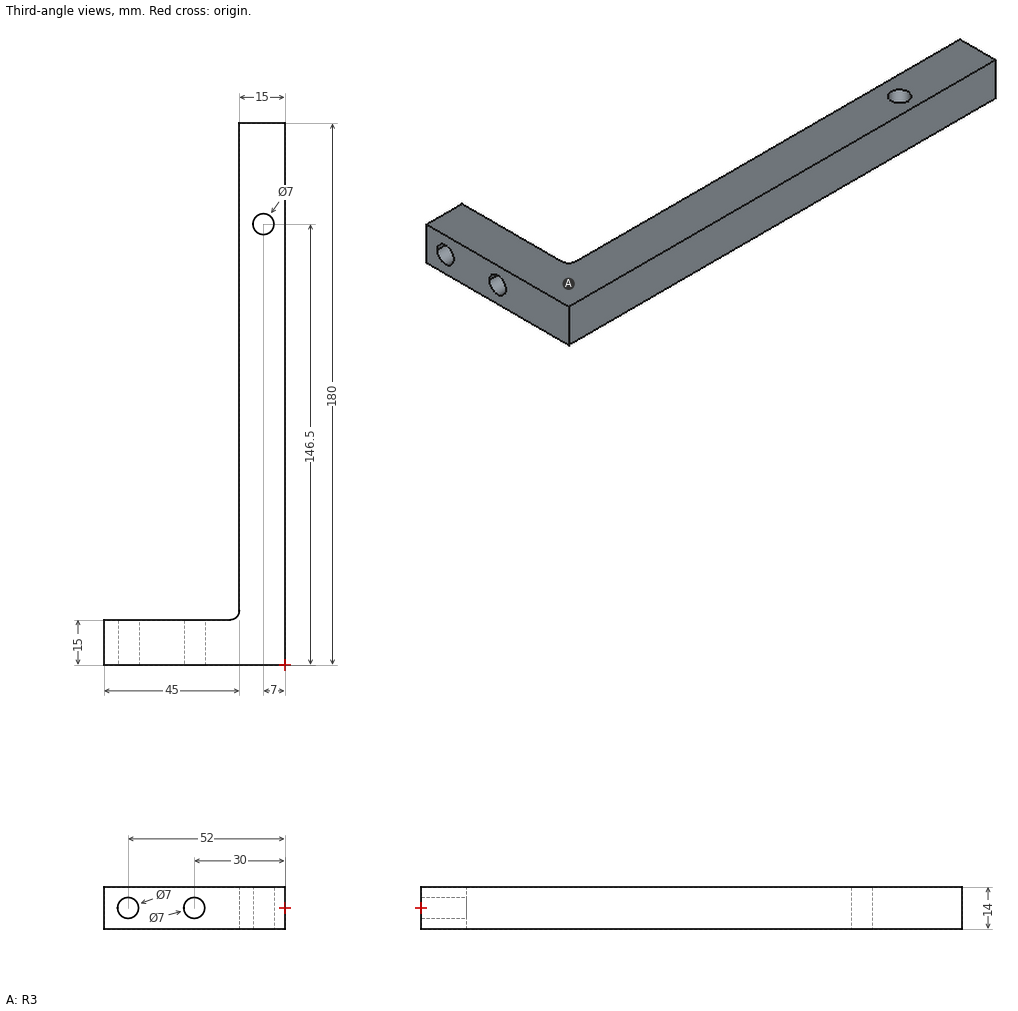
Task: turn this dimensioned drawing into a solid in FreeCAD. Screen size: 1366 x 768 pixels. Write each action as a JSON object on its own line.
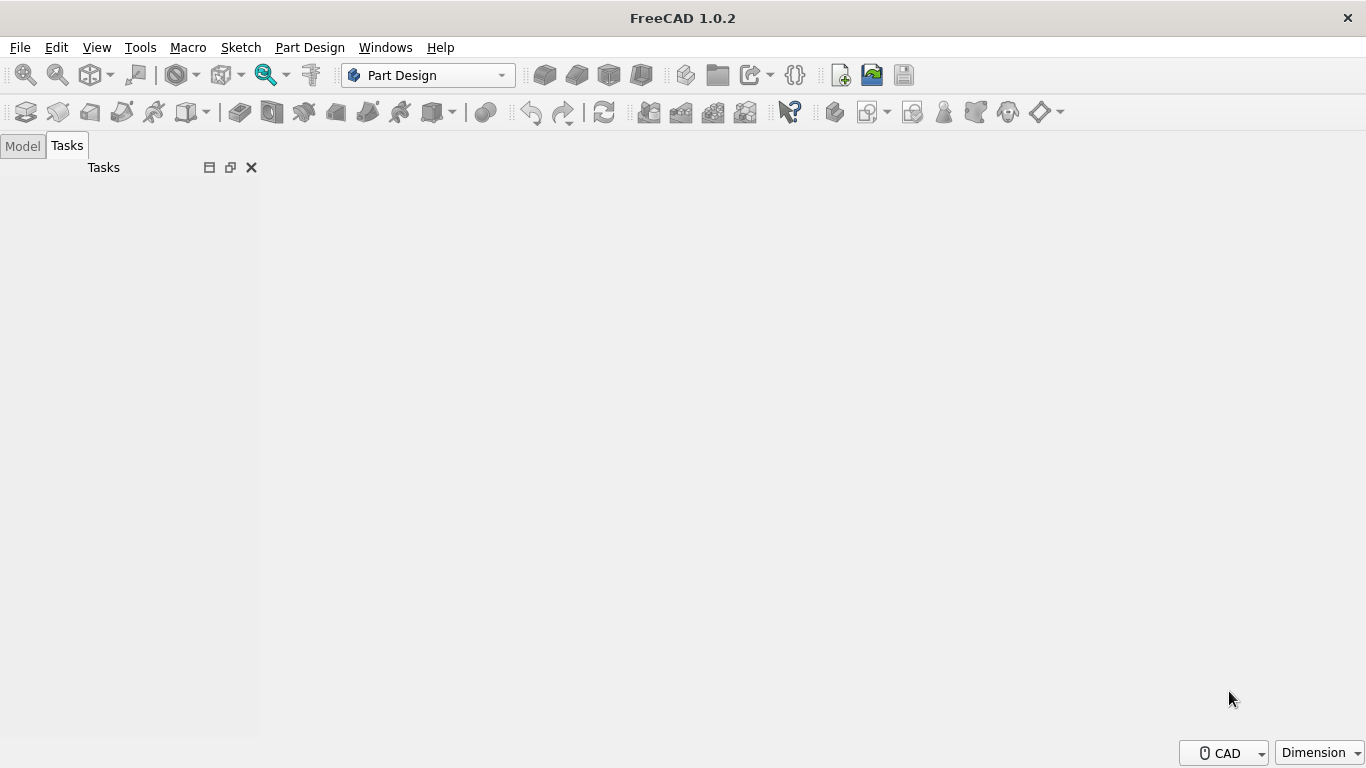
{"action": "left_click", "coordinate": [840, 76]}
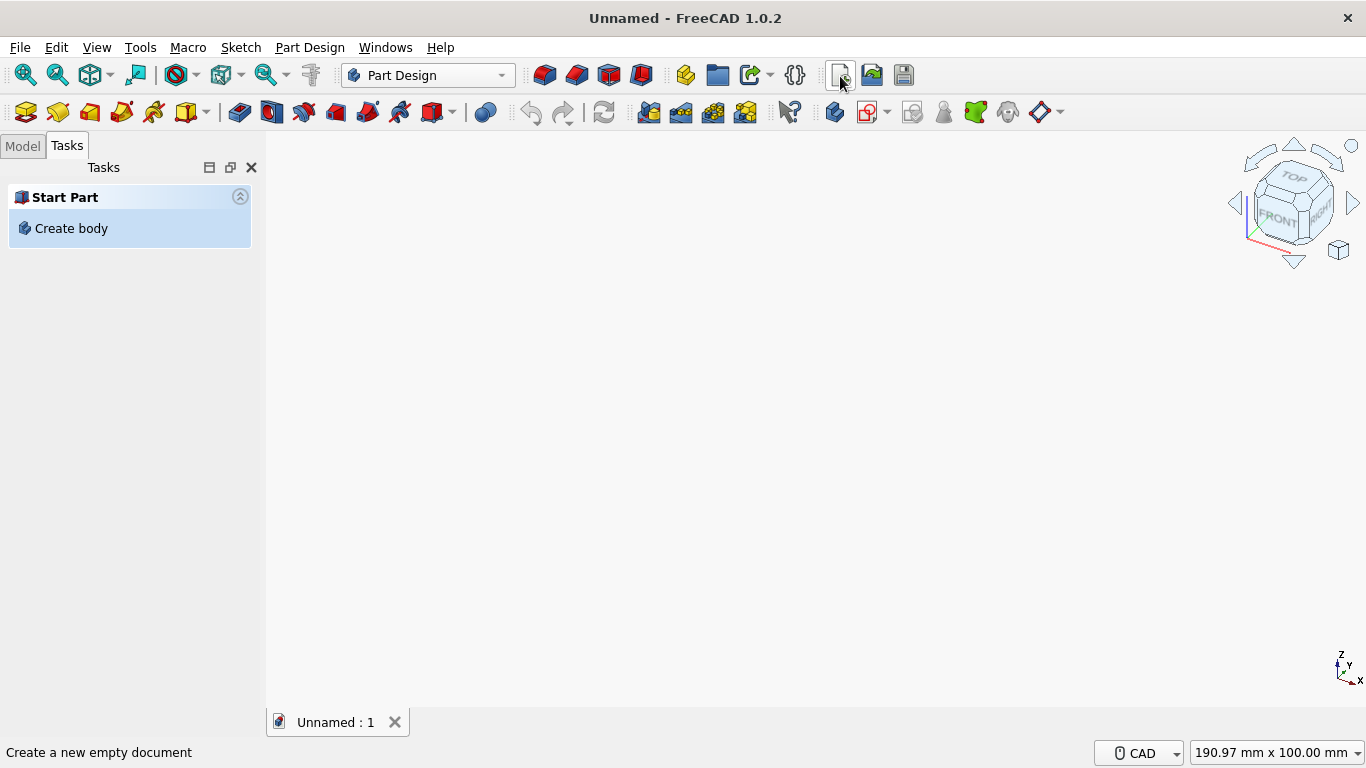
{"action": "left_click", "coordinate": [868, 112]}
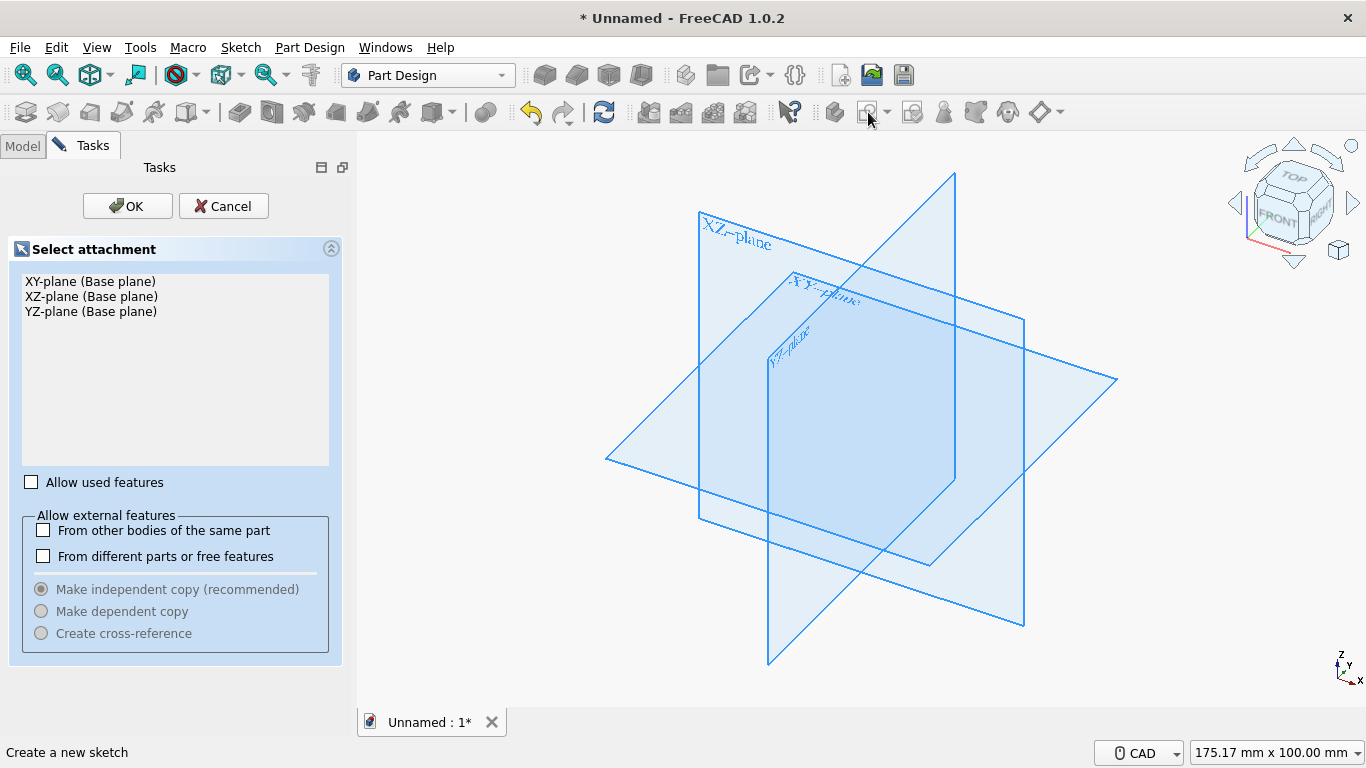
{"action": "left_click", "coordinate": [82, 282]}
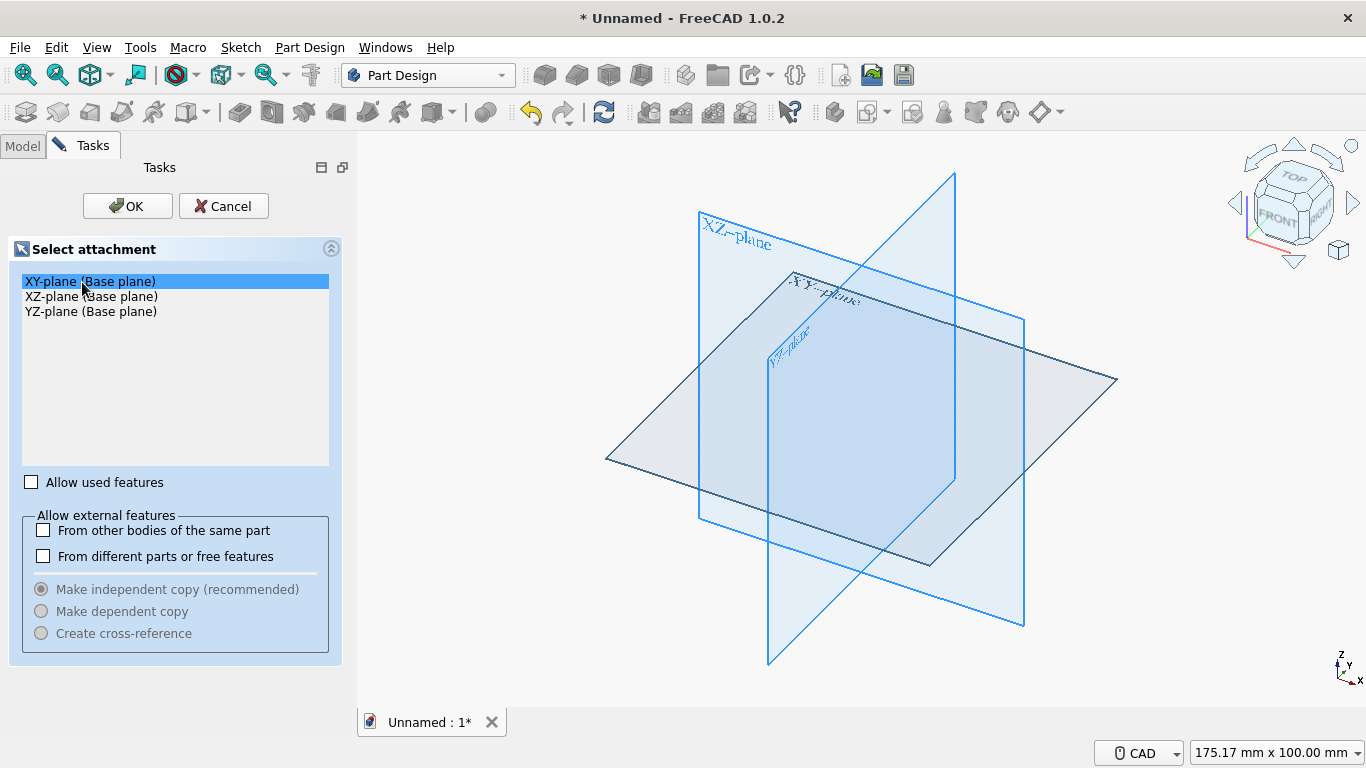
{"action": "left_click", "coordinate": [128, 206]}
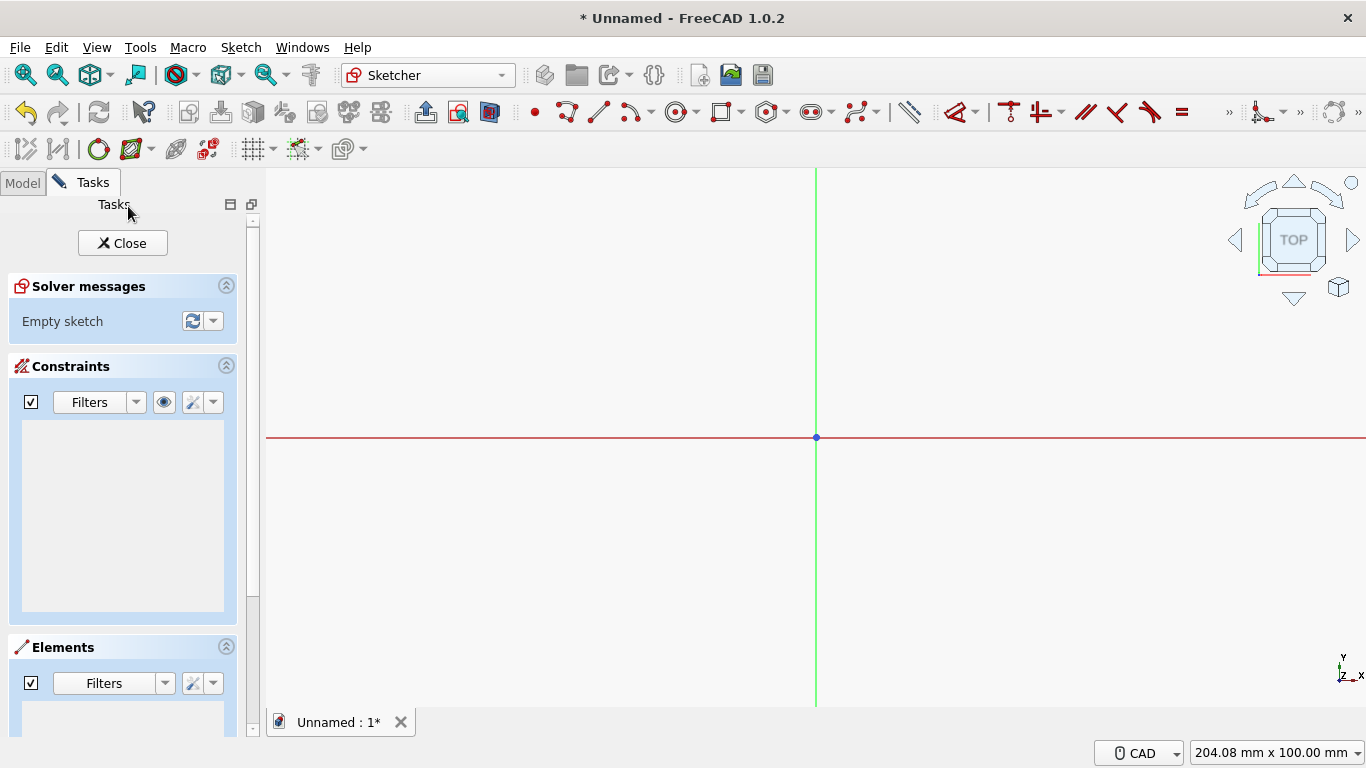
{"action": "scroll", "coordinate": [802, 679], "scroll_direction": "down", "scroll_amount": 5}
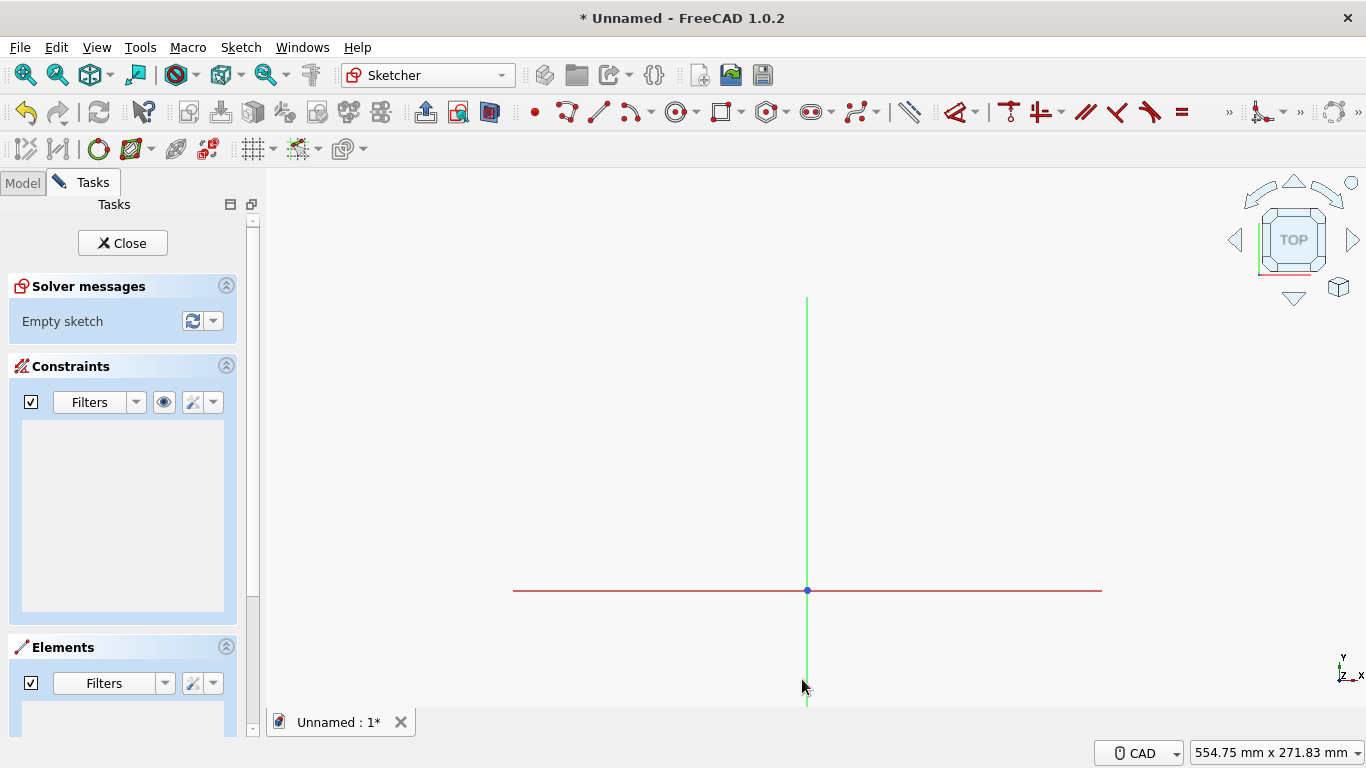
{"action": "left_click", "coordinate": [568, 112]}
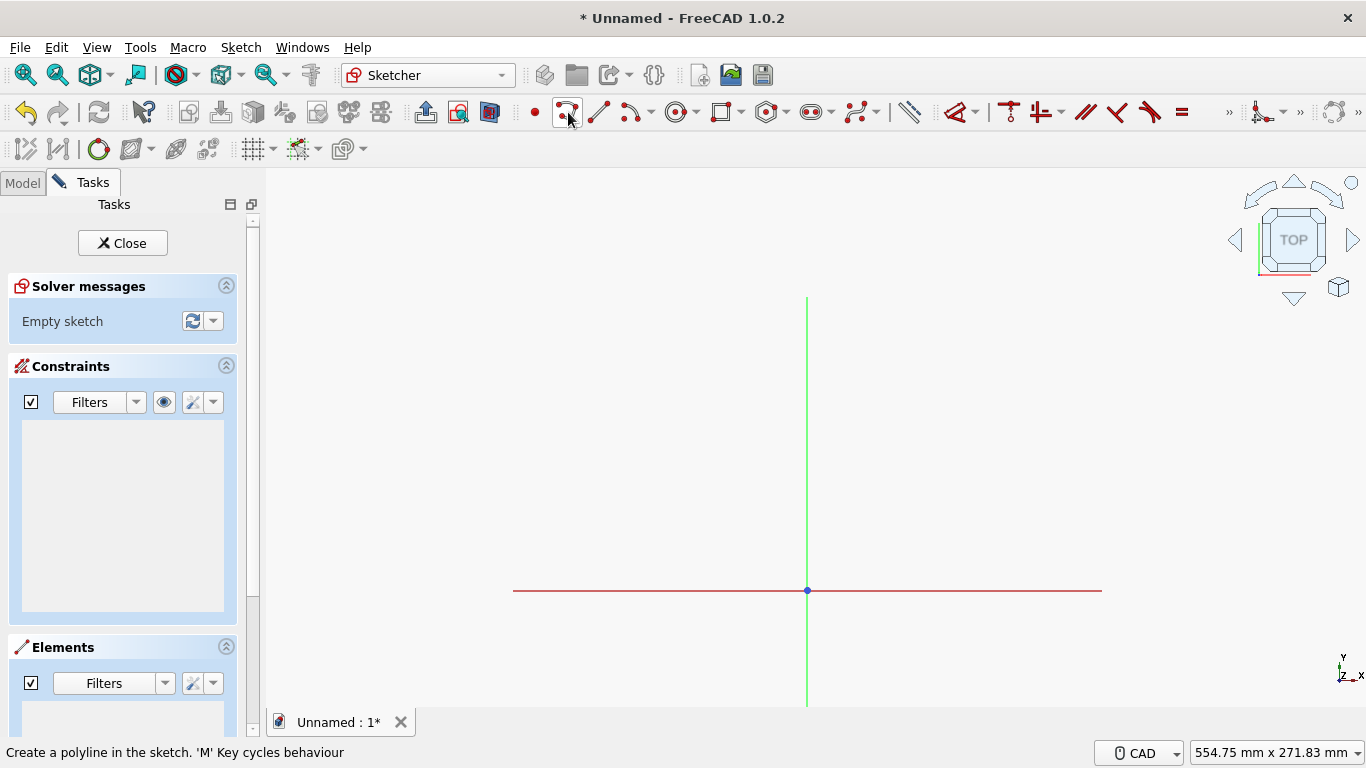
{"action": "left_click", "coordinate": [807, 591]}
{"action": "left_click", "coordinate": [798, 234]}
{"action": "left_click", "coordinate": [778, 234]}
{"action": "left_click", "coordinate": [778, 561]}
{"action": "left_click", "coordinate": [688, 561]}
{"action": "left_click", "coordinate": [688, 582]}
{"action": "left_click", "coordinate": [807, 591]}
{"action": "key", "text": "Escape"}
{"action": "key", "text": "Escape"}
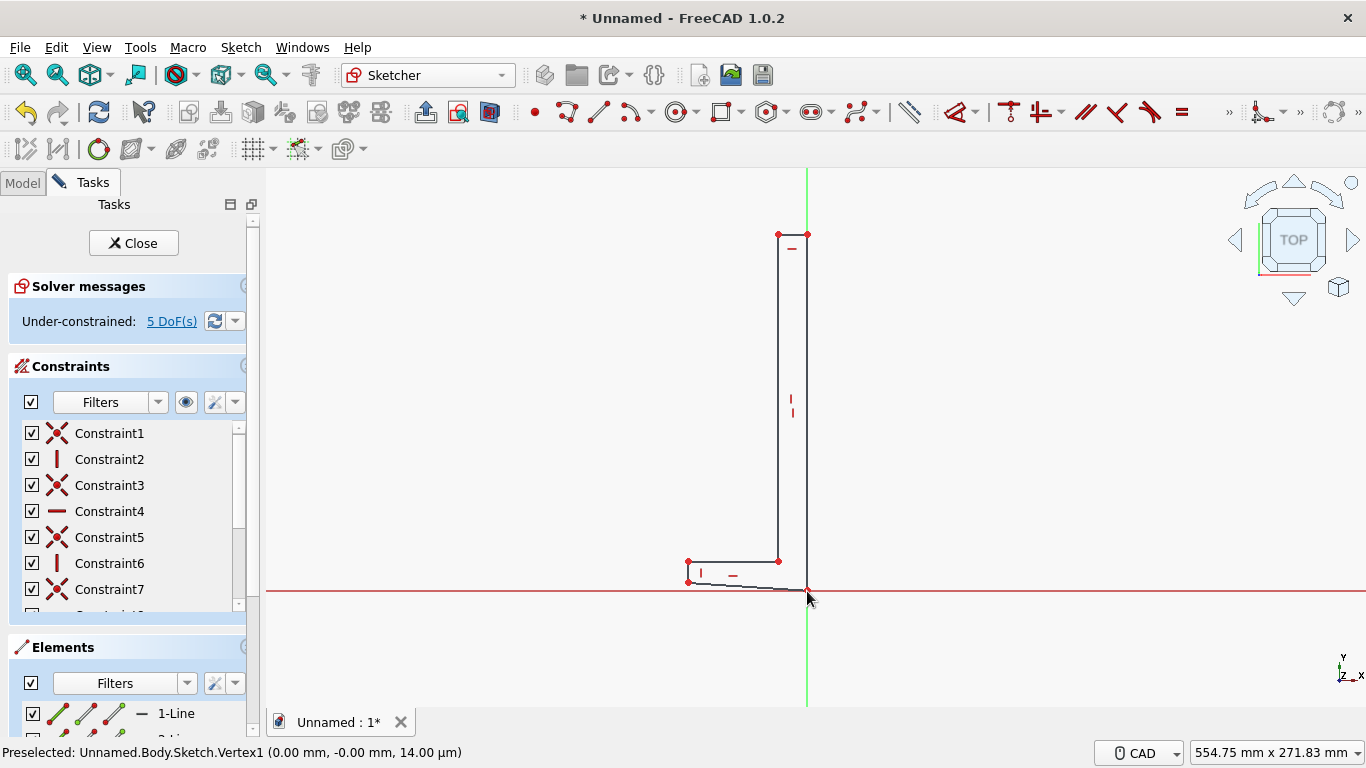
{"action": "left_click", "coordinate": [772, 588]}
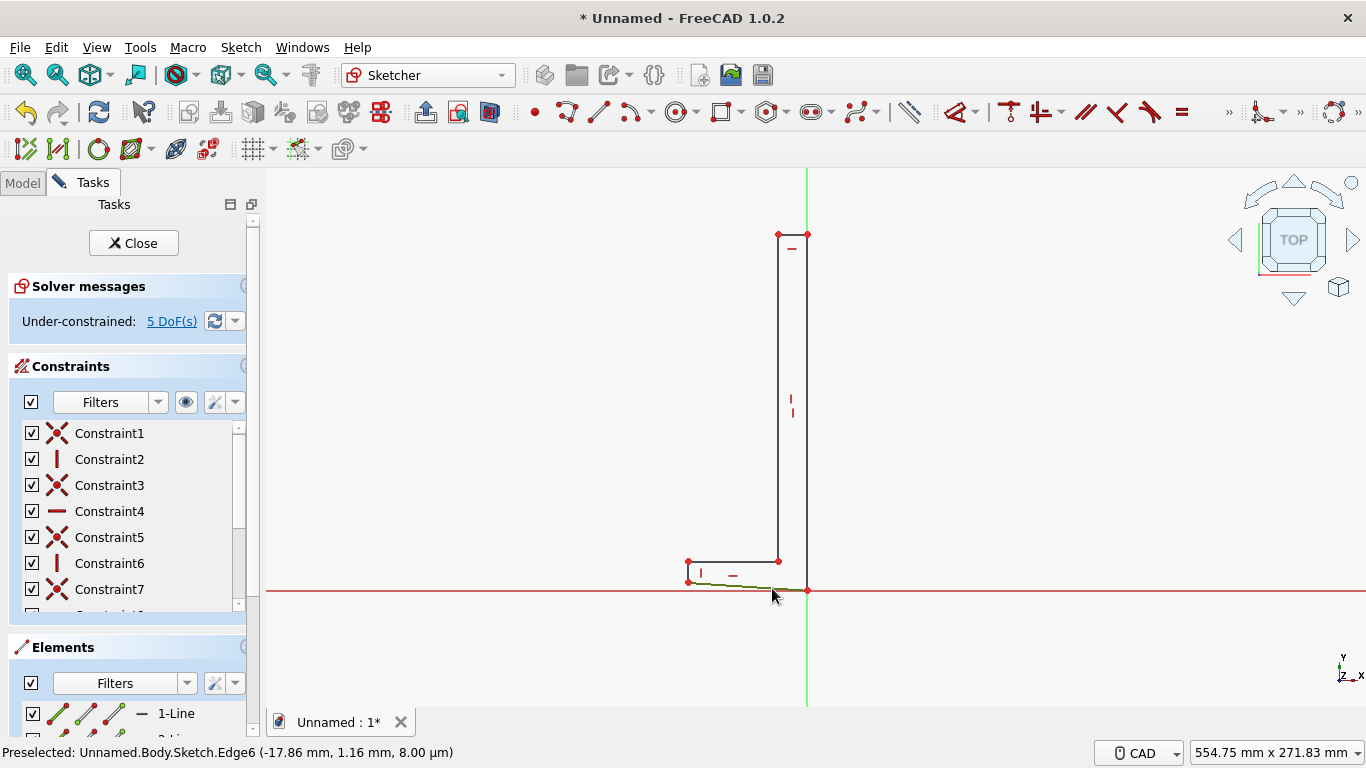
{"action": "key", "text": "h"}